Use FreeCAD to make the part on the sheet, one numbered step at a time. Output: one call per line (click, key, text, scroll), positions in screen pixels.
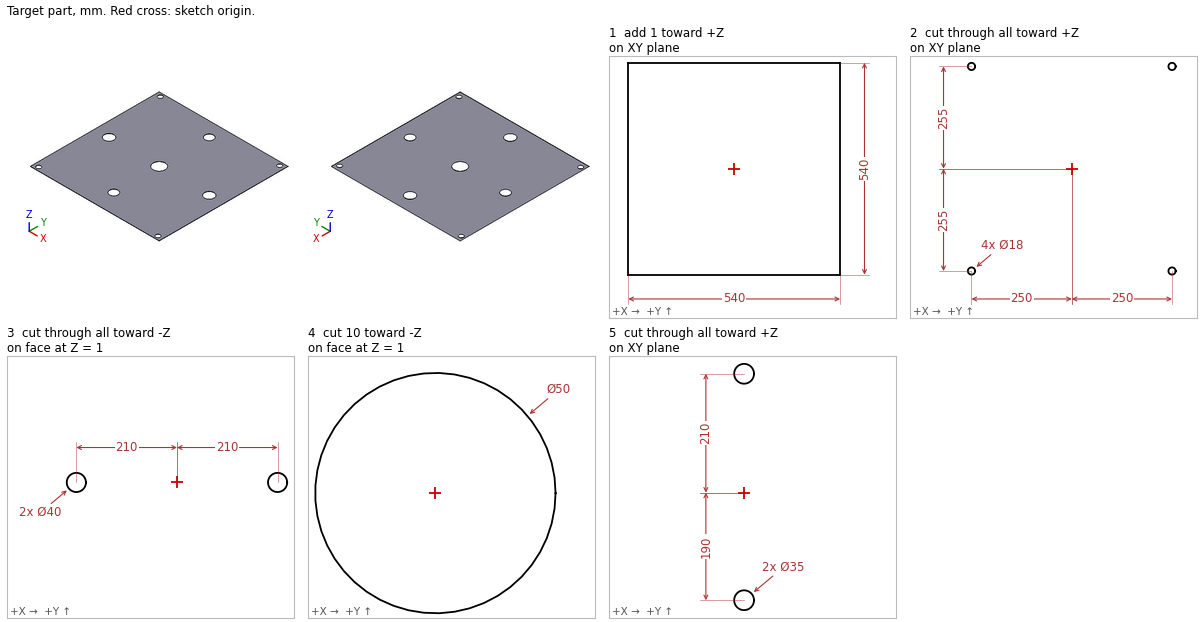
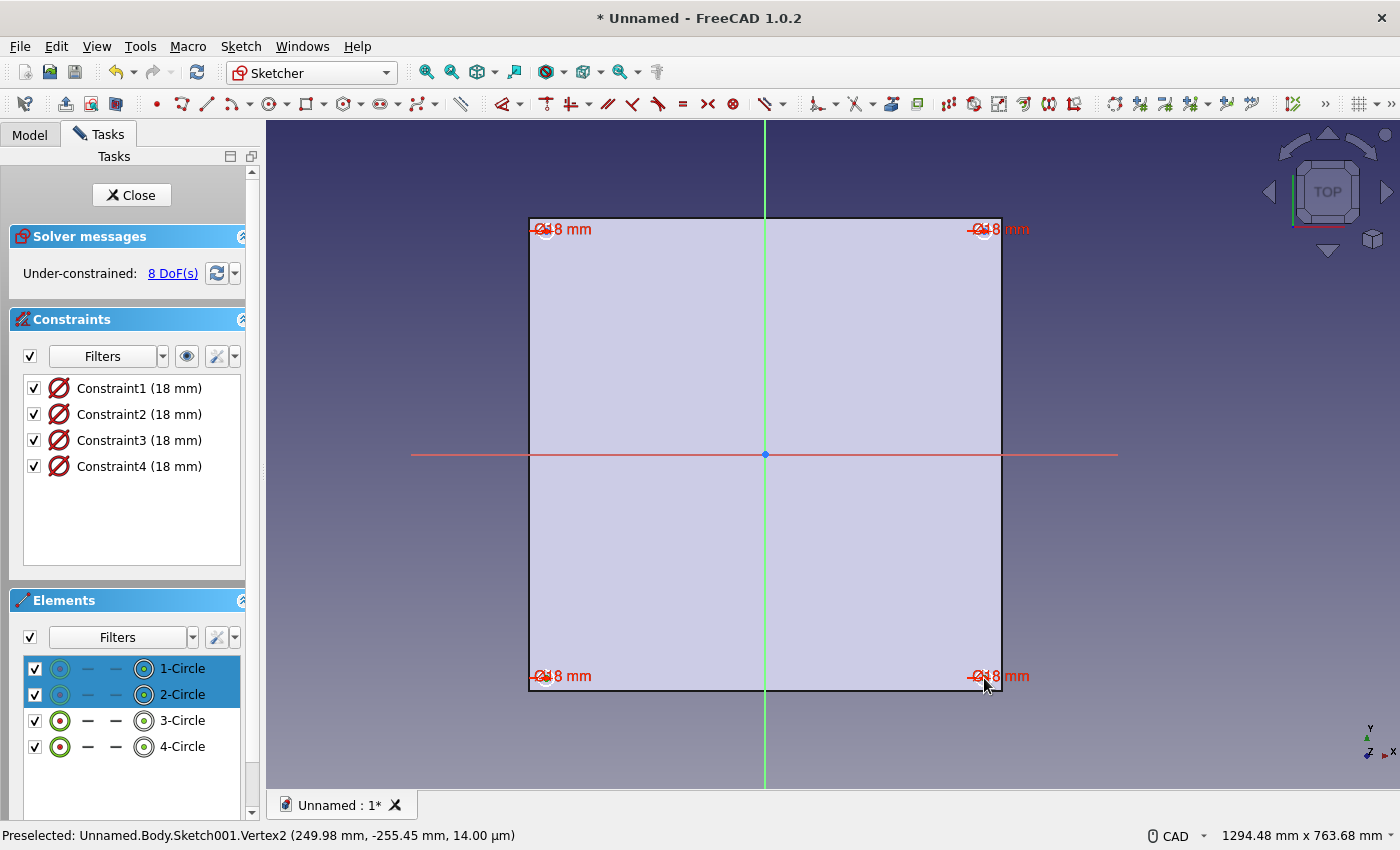
click(588, 104)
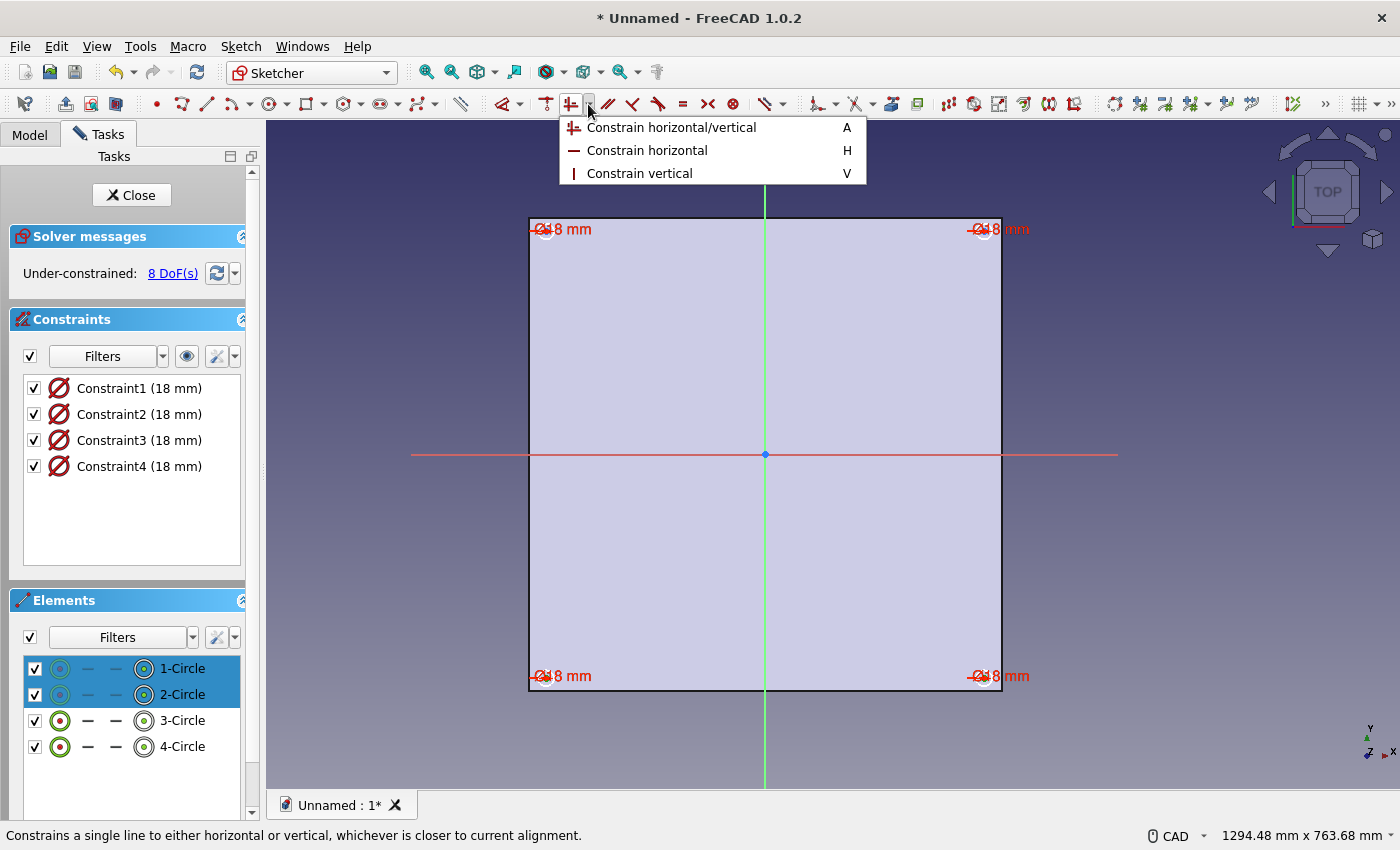
click(713, 150)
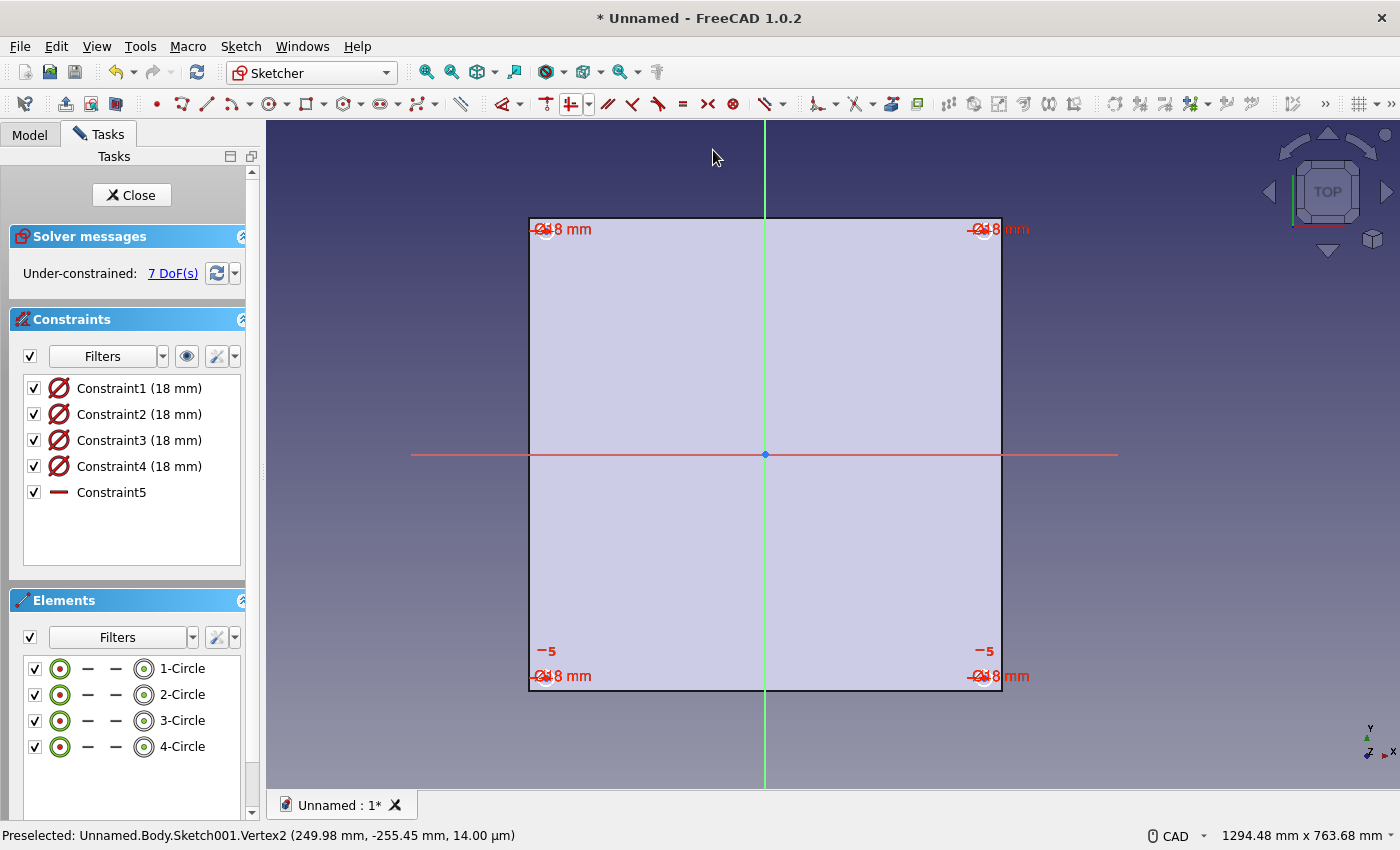
click(546, 678)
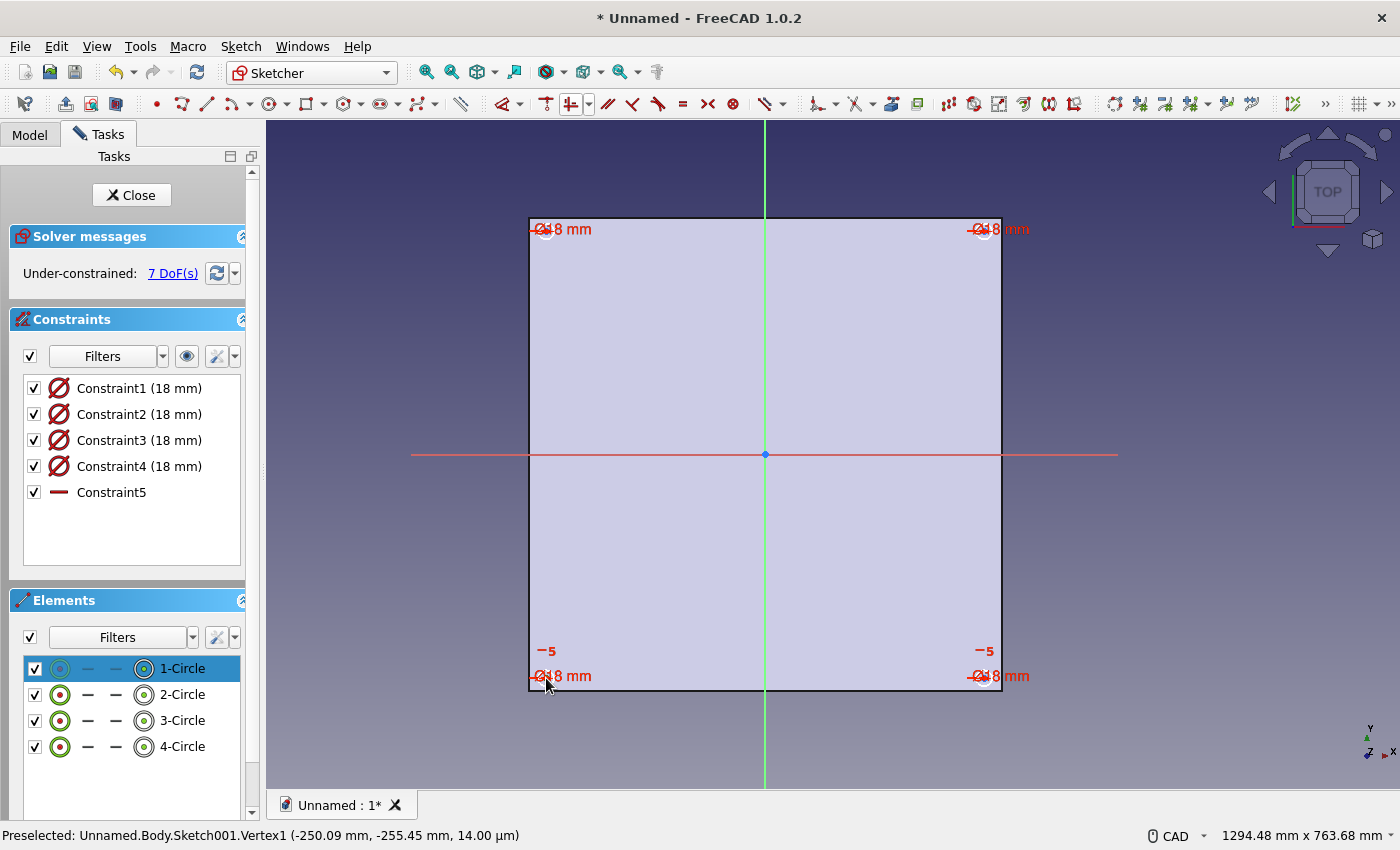
click(546, 231)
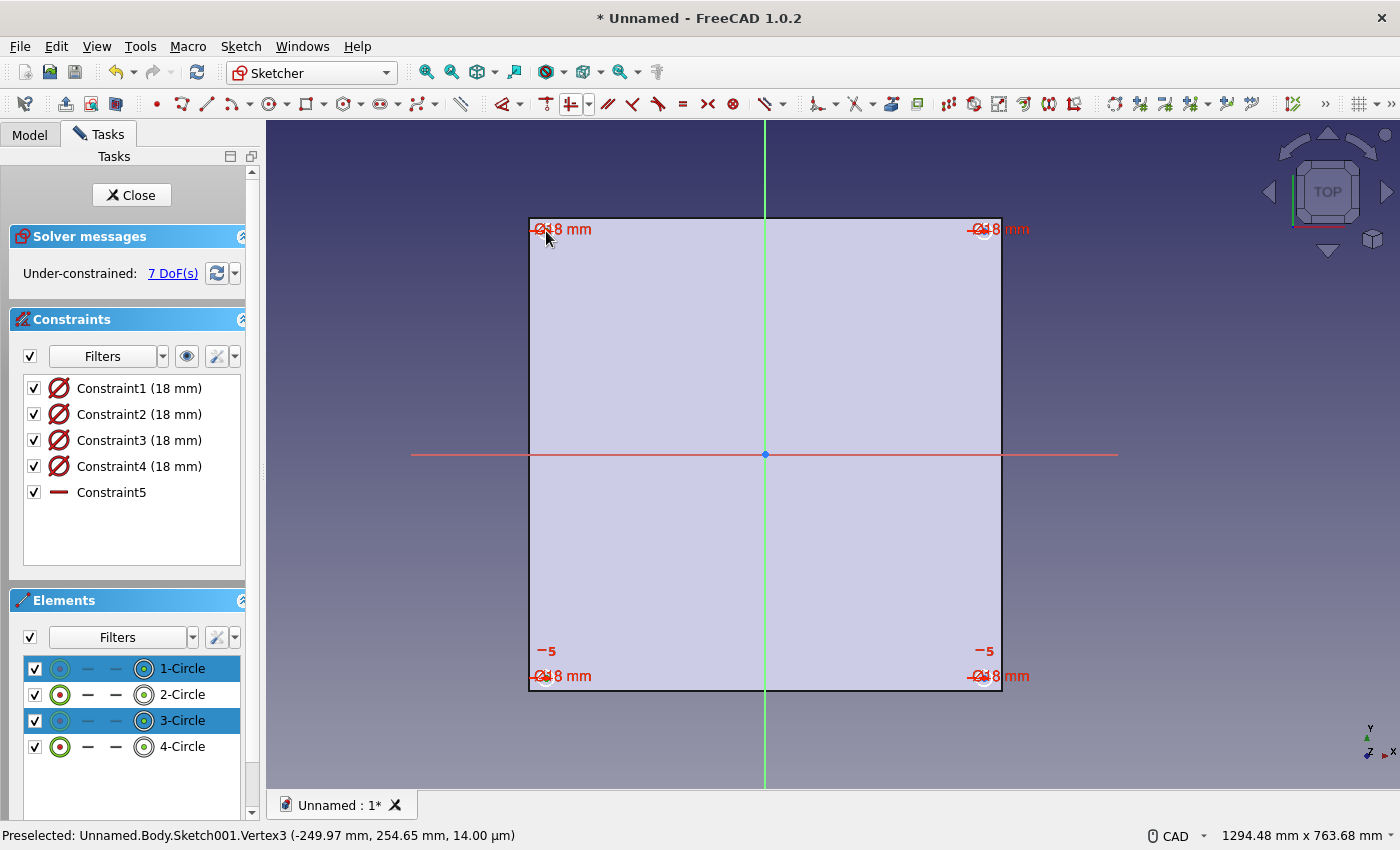
key(v)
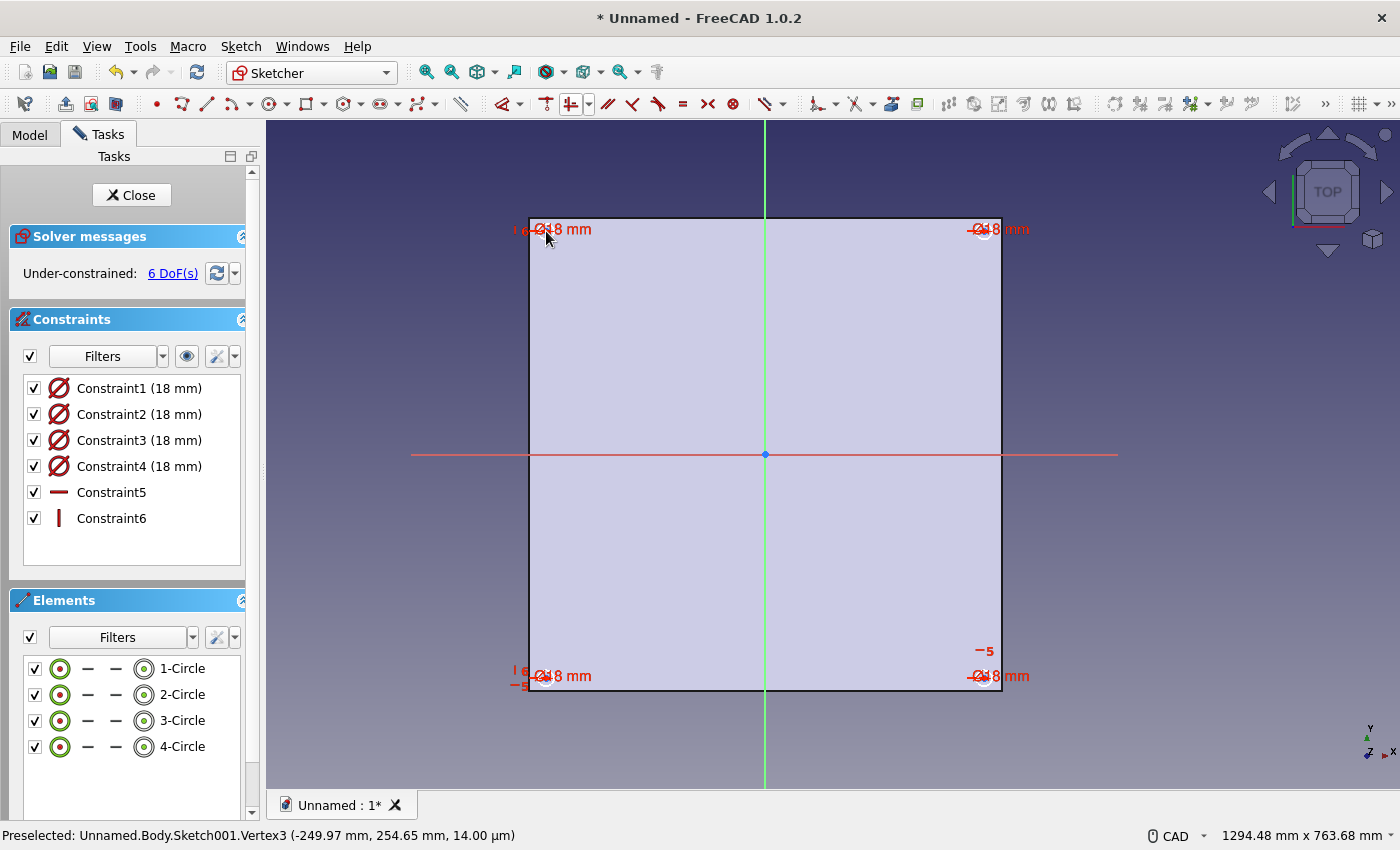
click(984, 678)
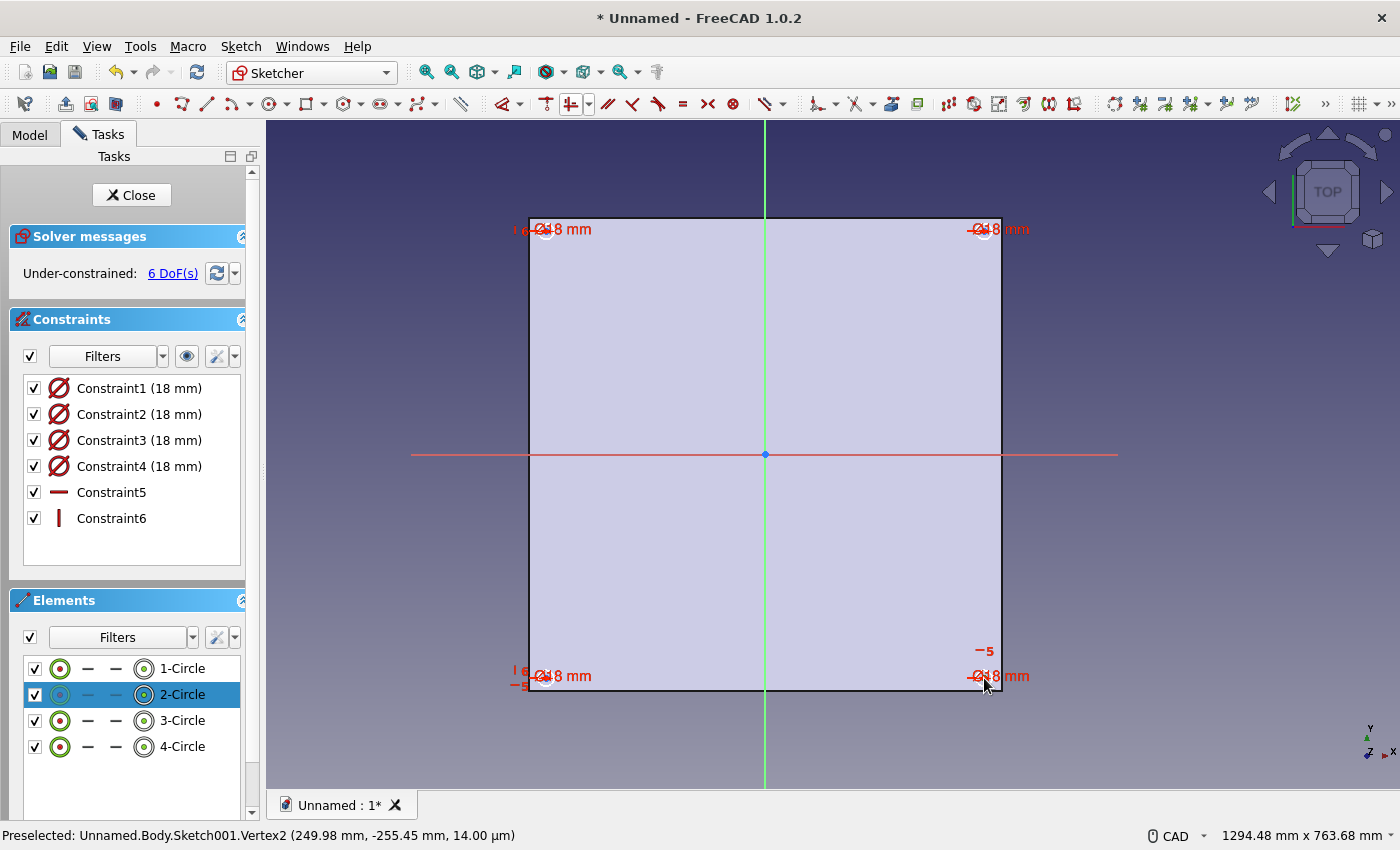
click(984, 231)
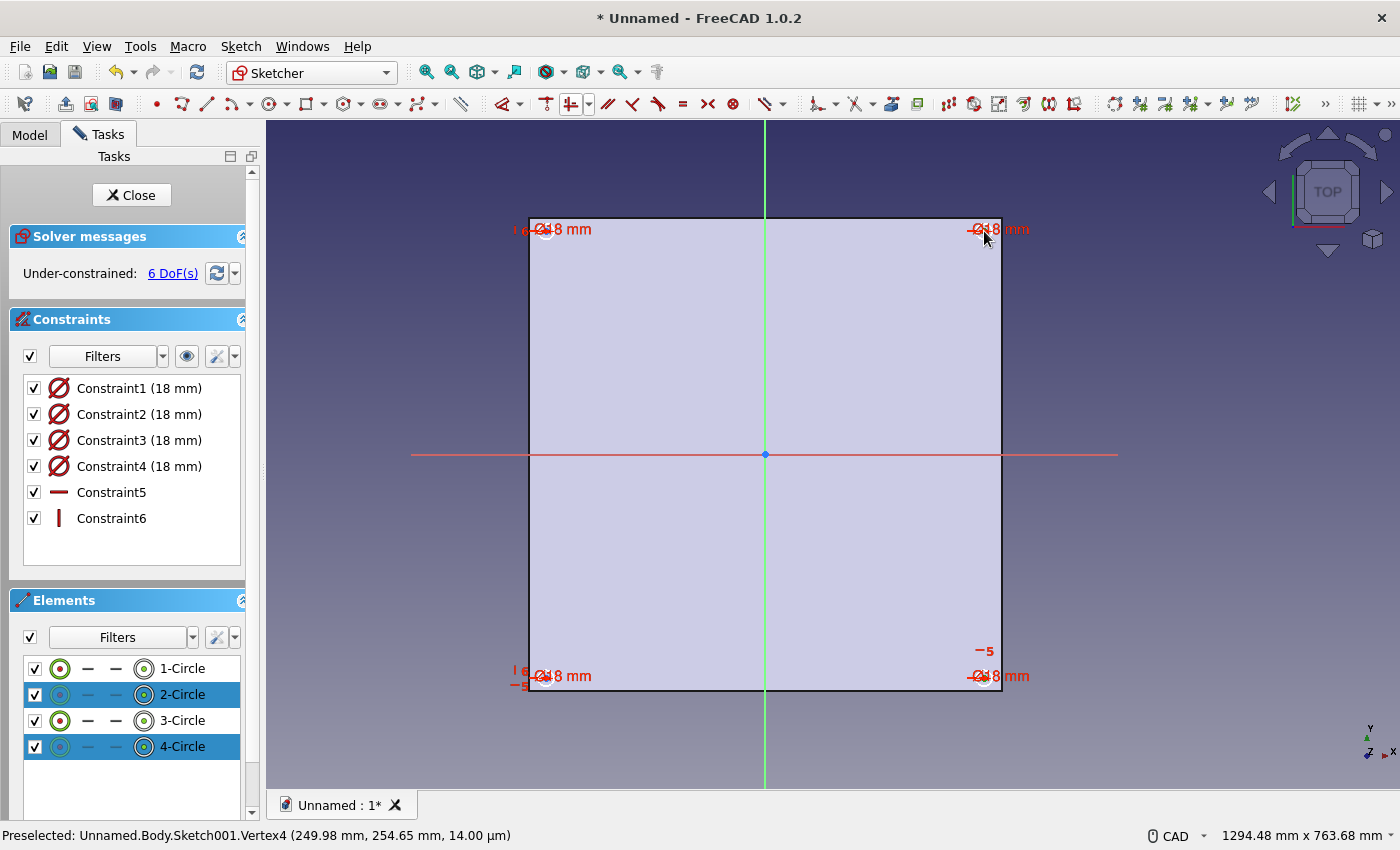
key(v)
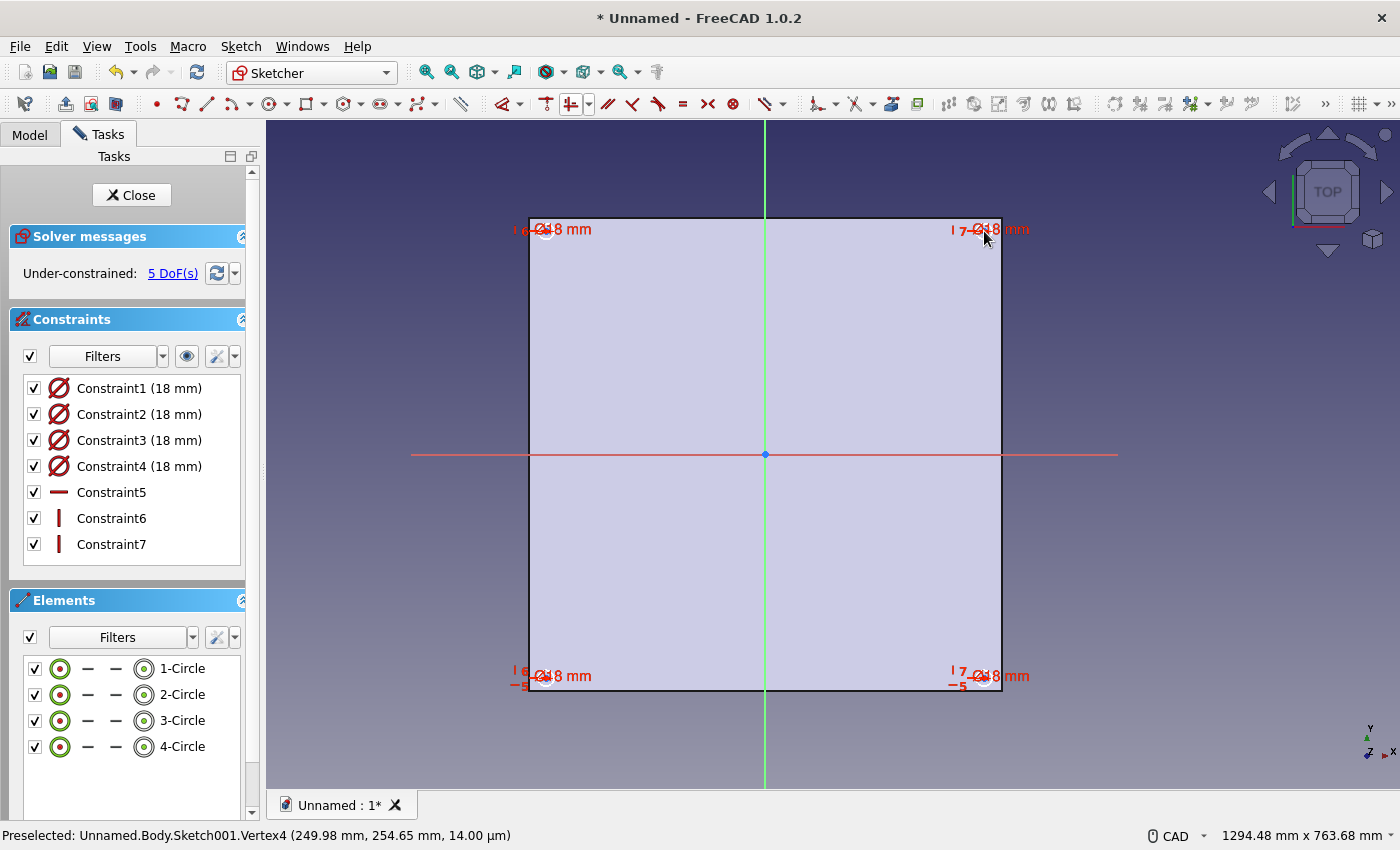
click(546, 231)